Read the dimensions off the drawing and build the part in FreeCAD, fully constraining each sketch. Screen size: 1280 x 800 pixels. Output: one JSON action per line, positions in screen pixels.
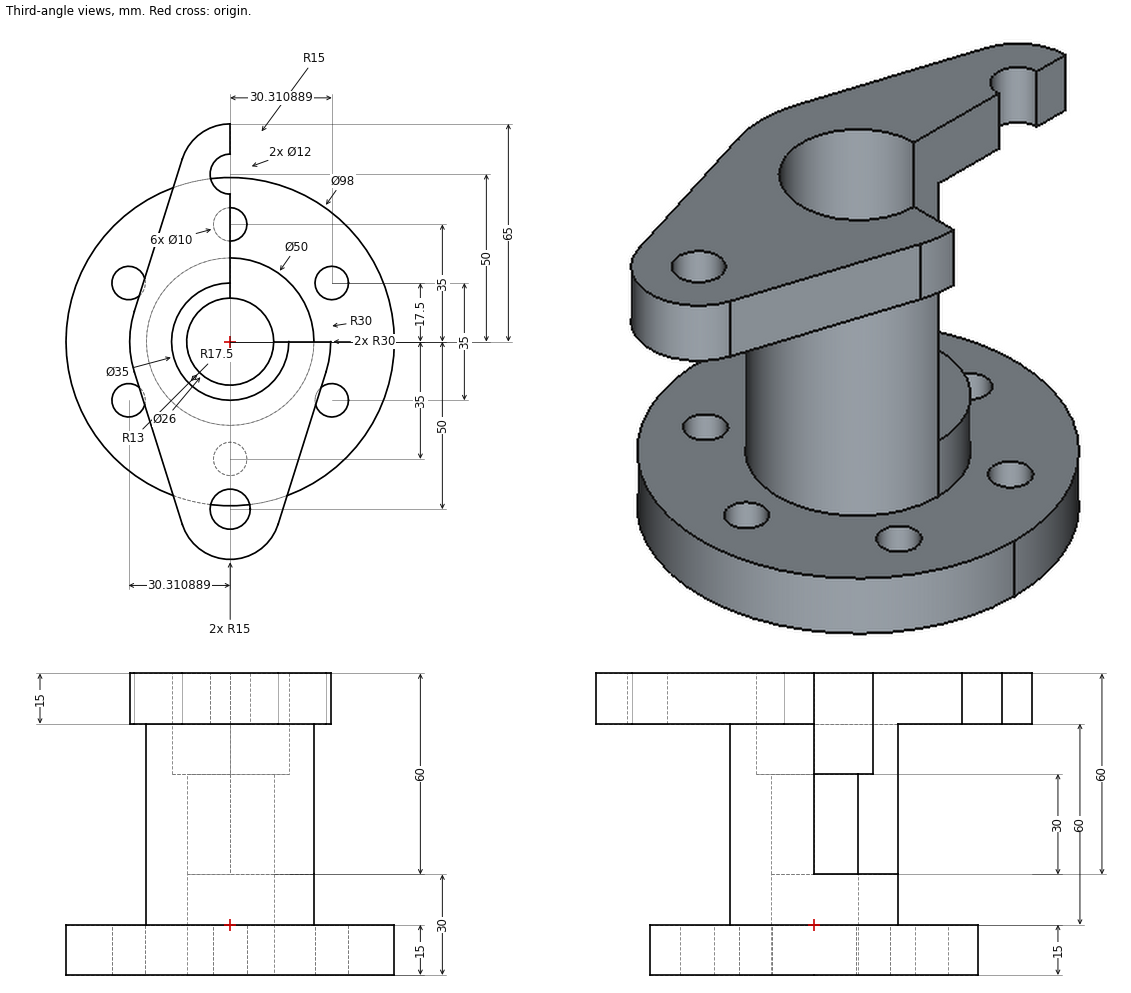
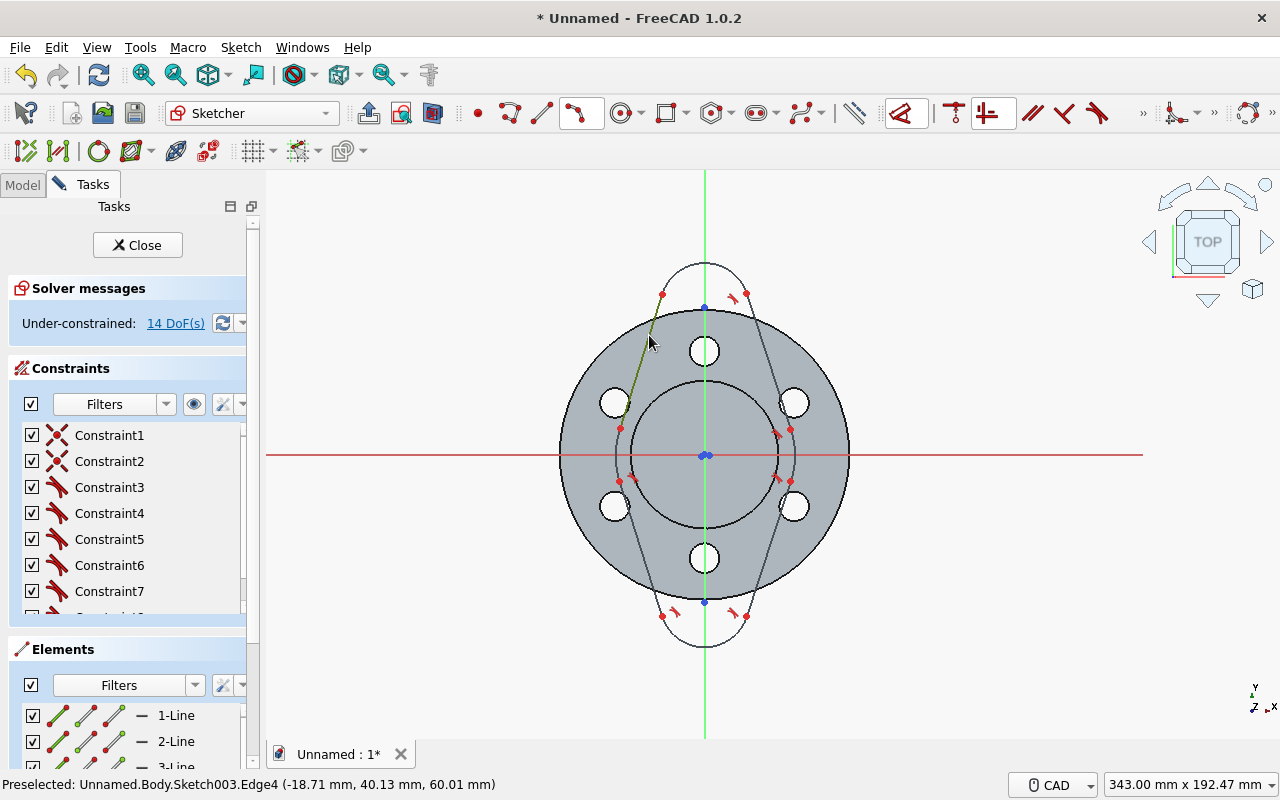
{"action": "left_click", "coordinate": [726, 268]}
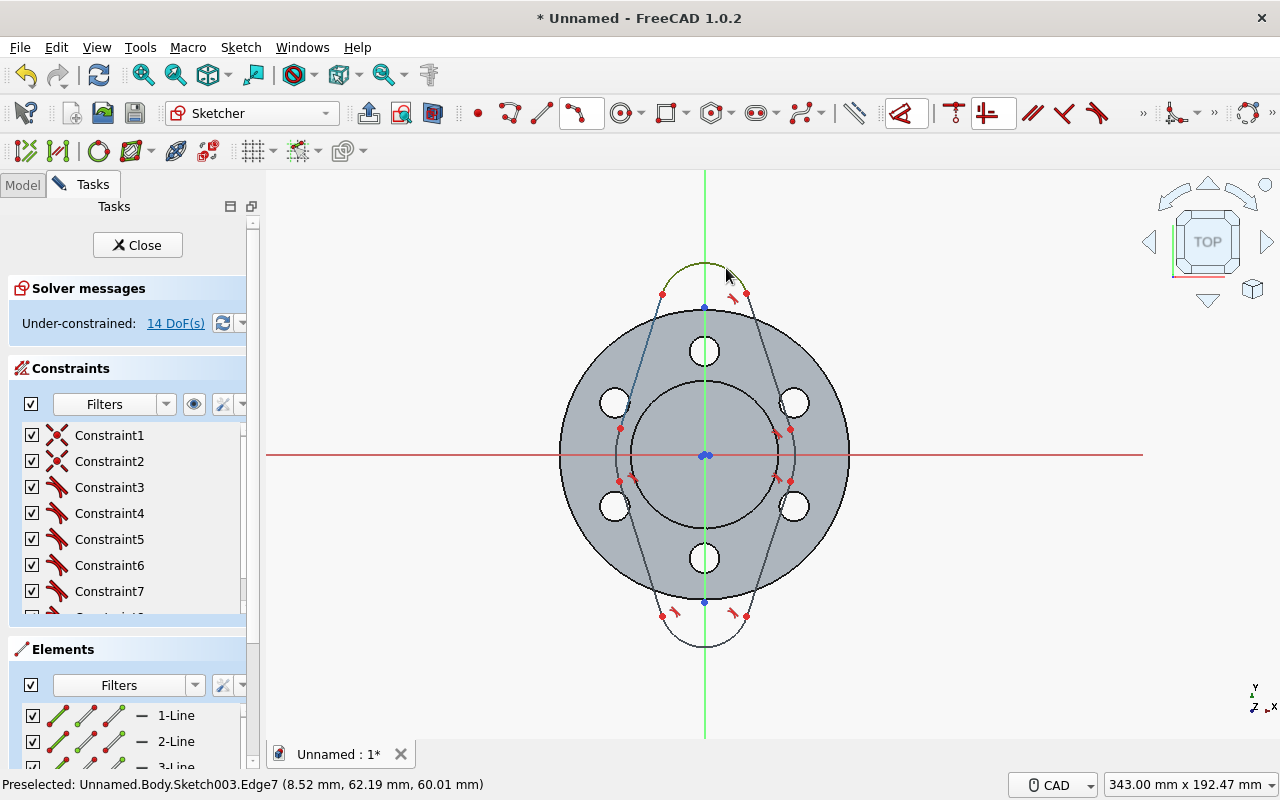
{"action": "left_click", "coordinate": [1098, 114]}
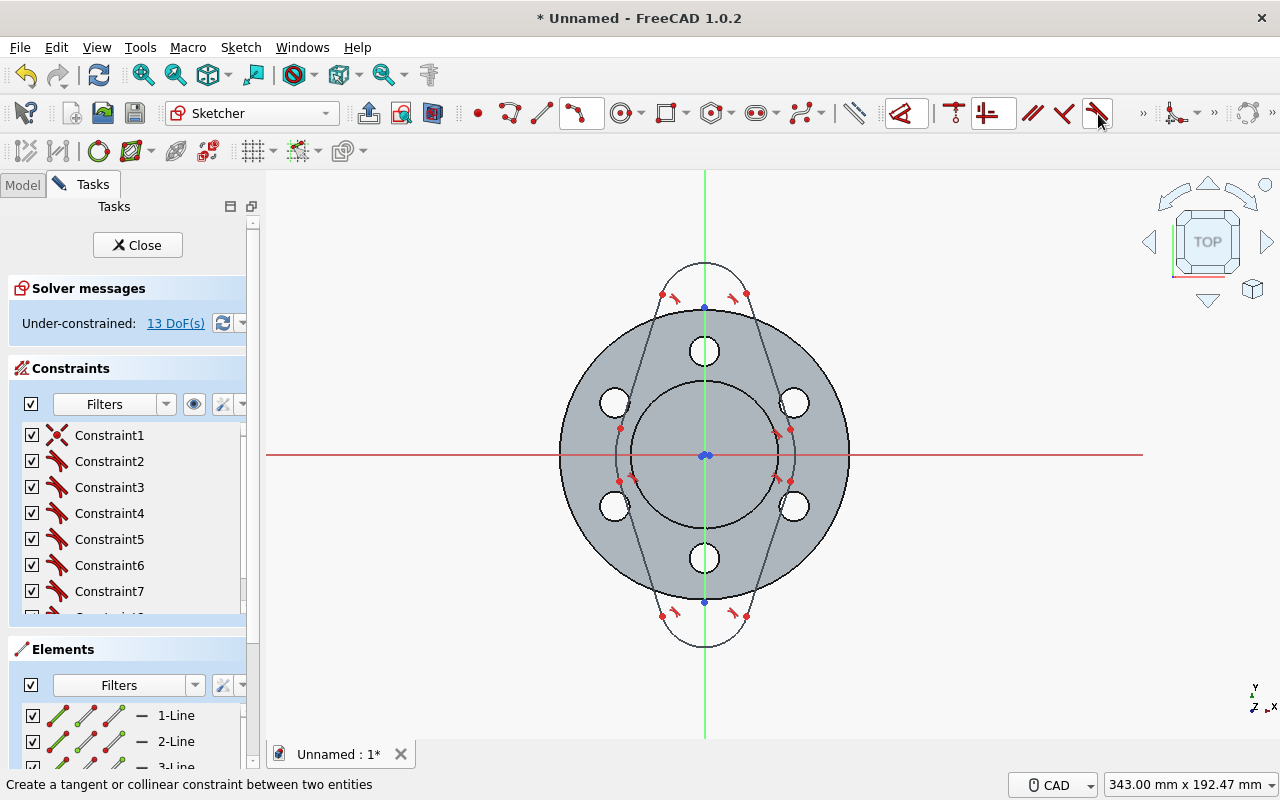
{"action": "left_click", "coordinate": [649, 335]}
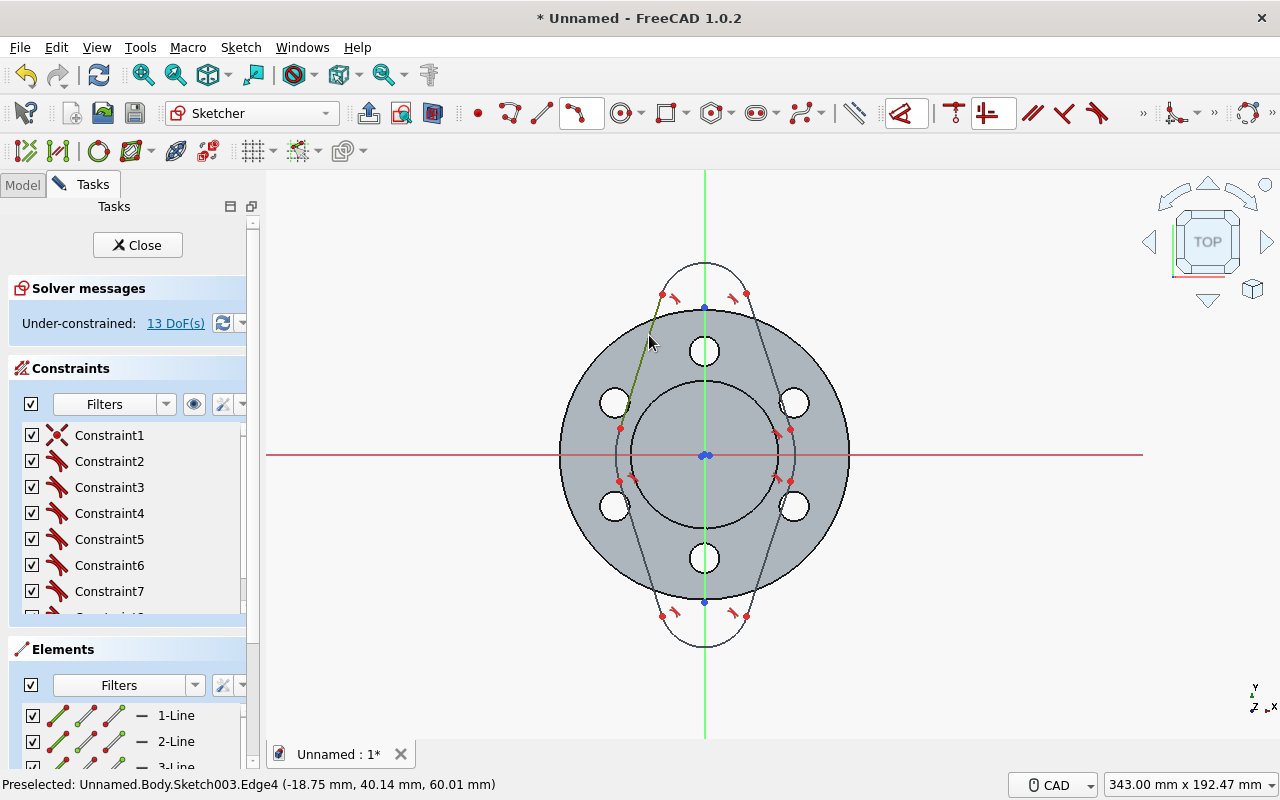
{"action": "scroll", "coordinate": [617, 445], "scroll_direction": "up", "scroll_amount": 2}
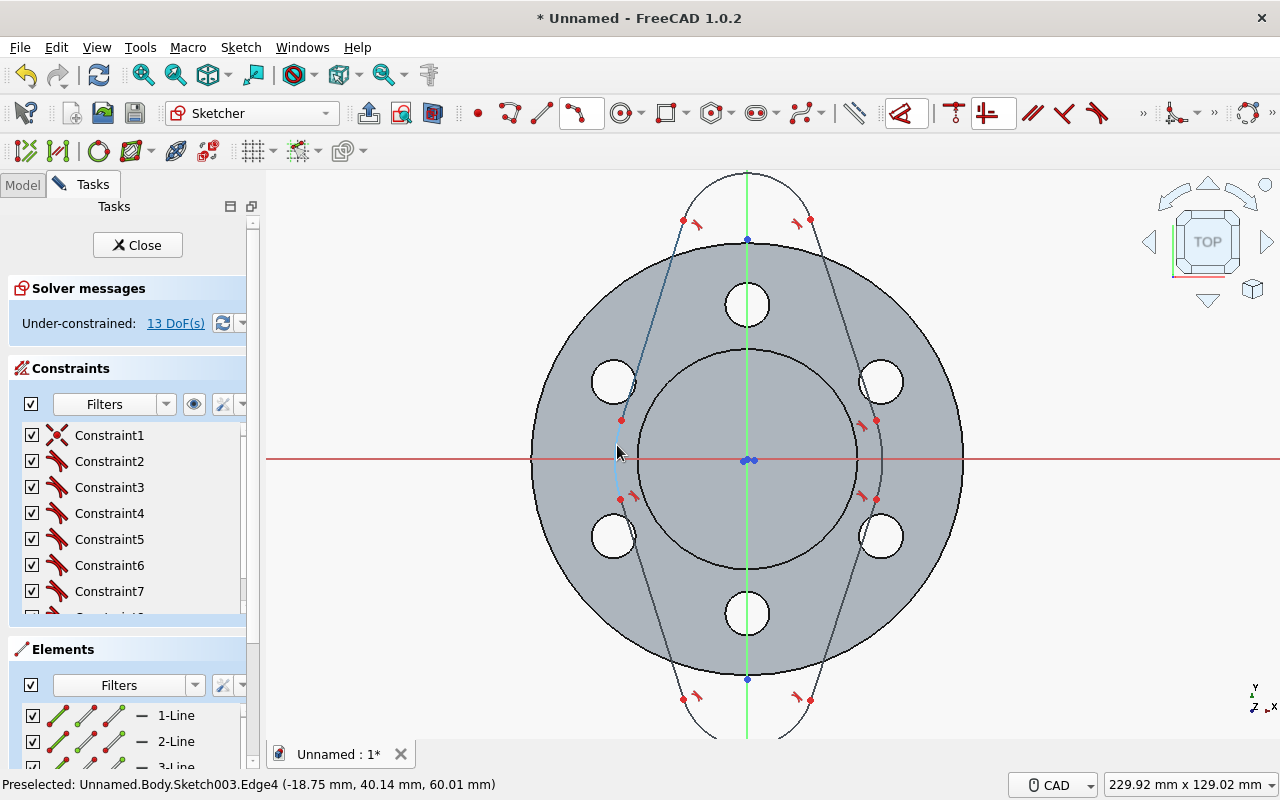
{"action": "left_click", "coordinate": [616, 444]}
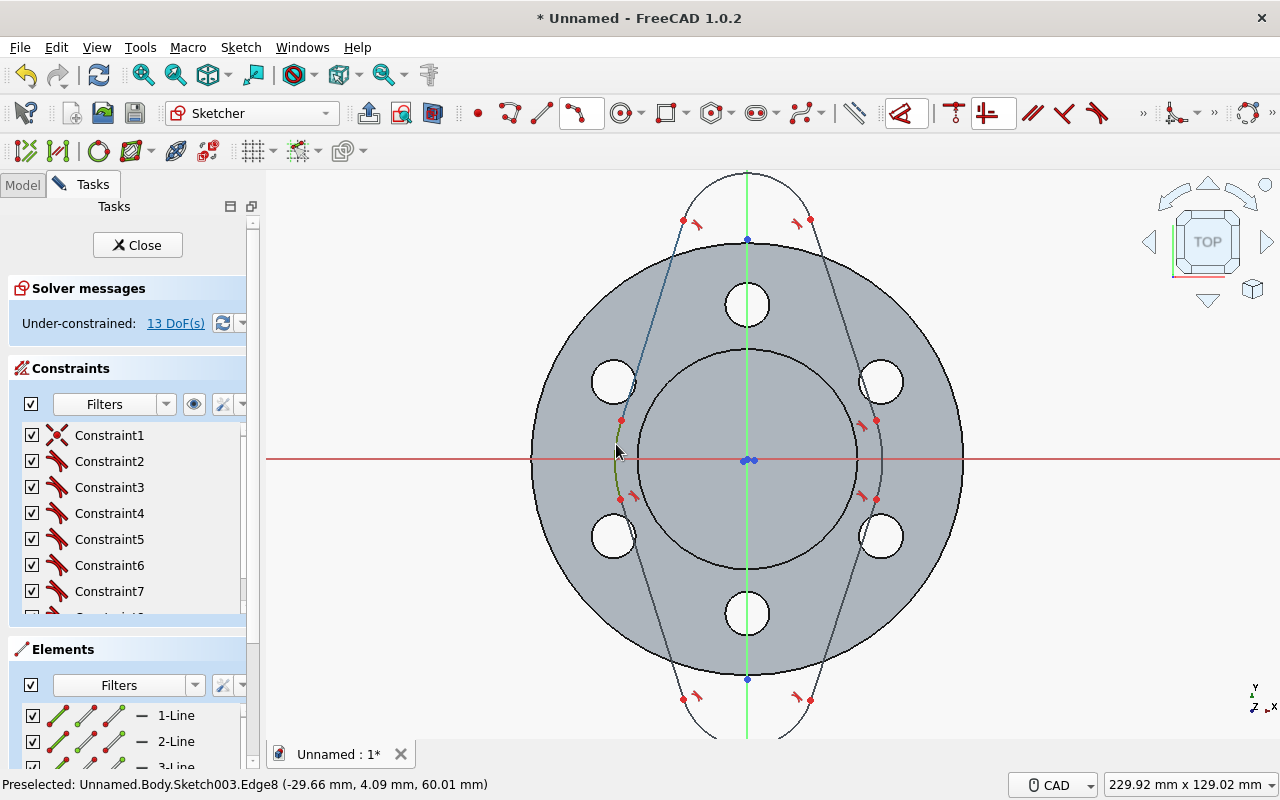
{"action": "left_click", "coordinate": [1098, 114]}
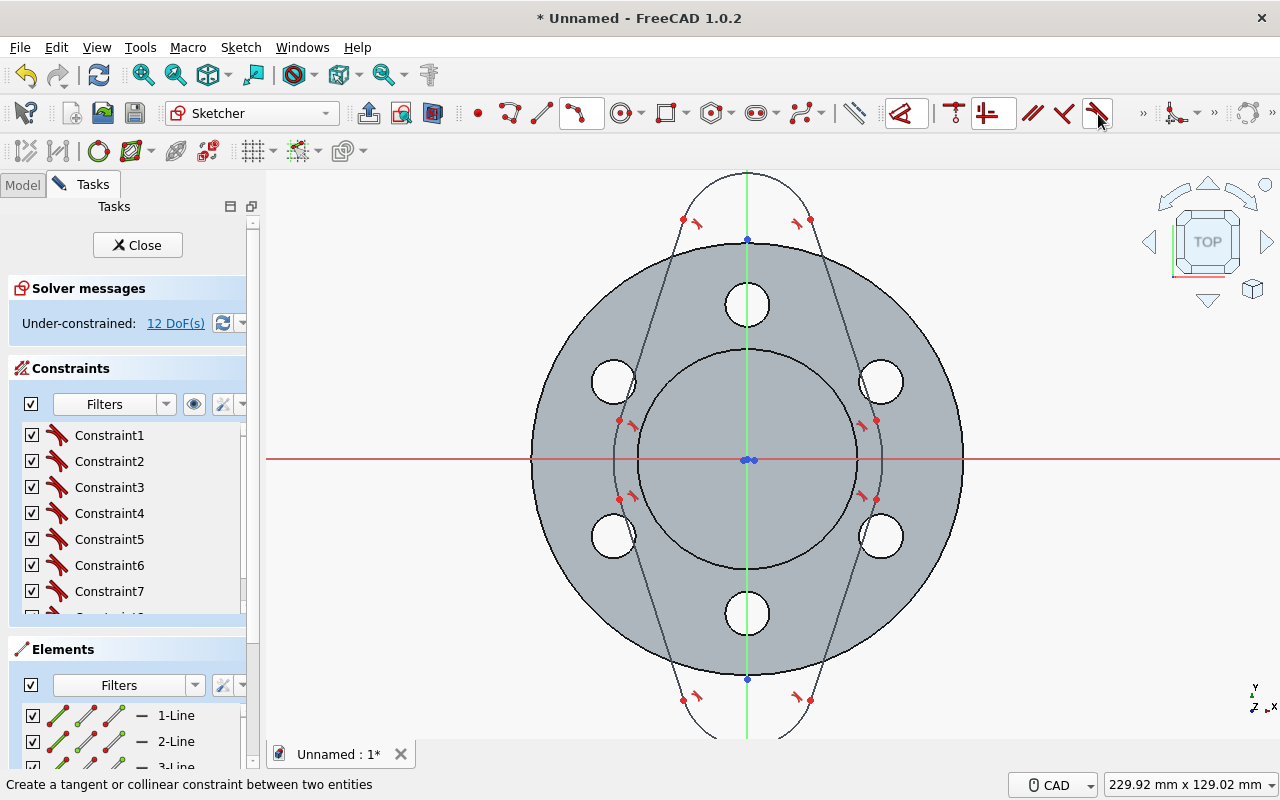
{"action": "left_click", "coordinate": [881, 476]}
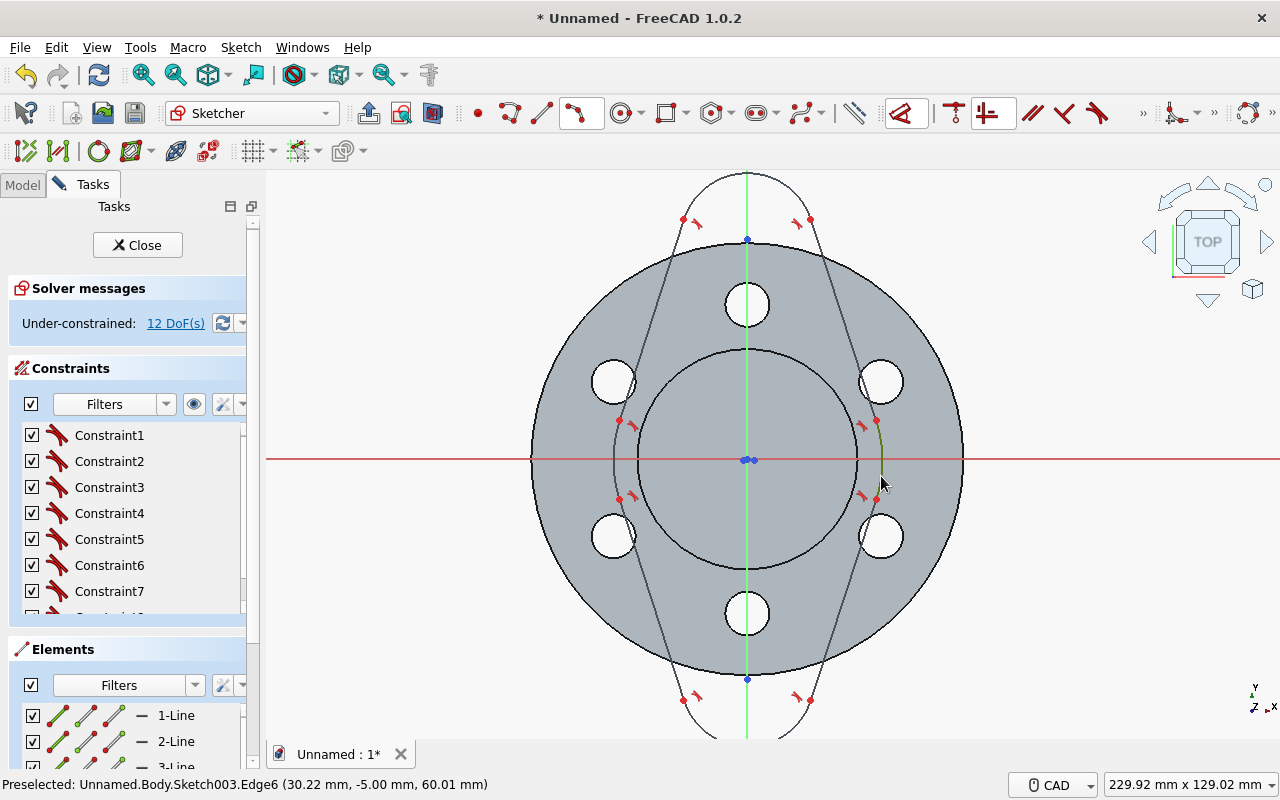
{"action": "left_click", "coordinate": [615, 444]}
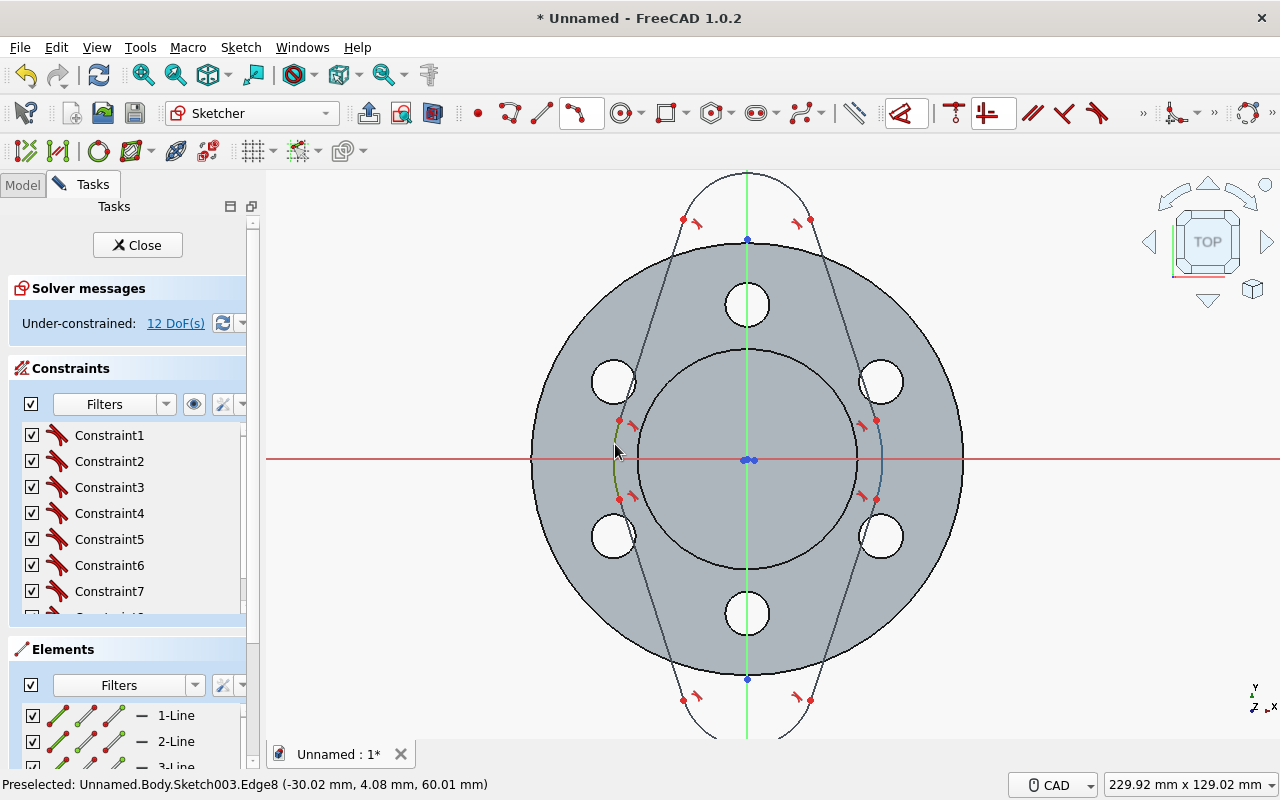
{"action": "left_click", "coordinate": [954, 114]}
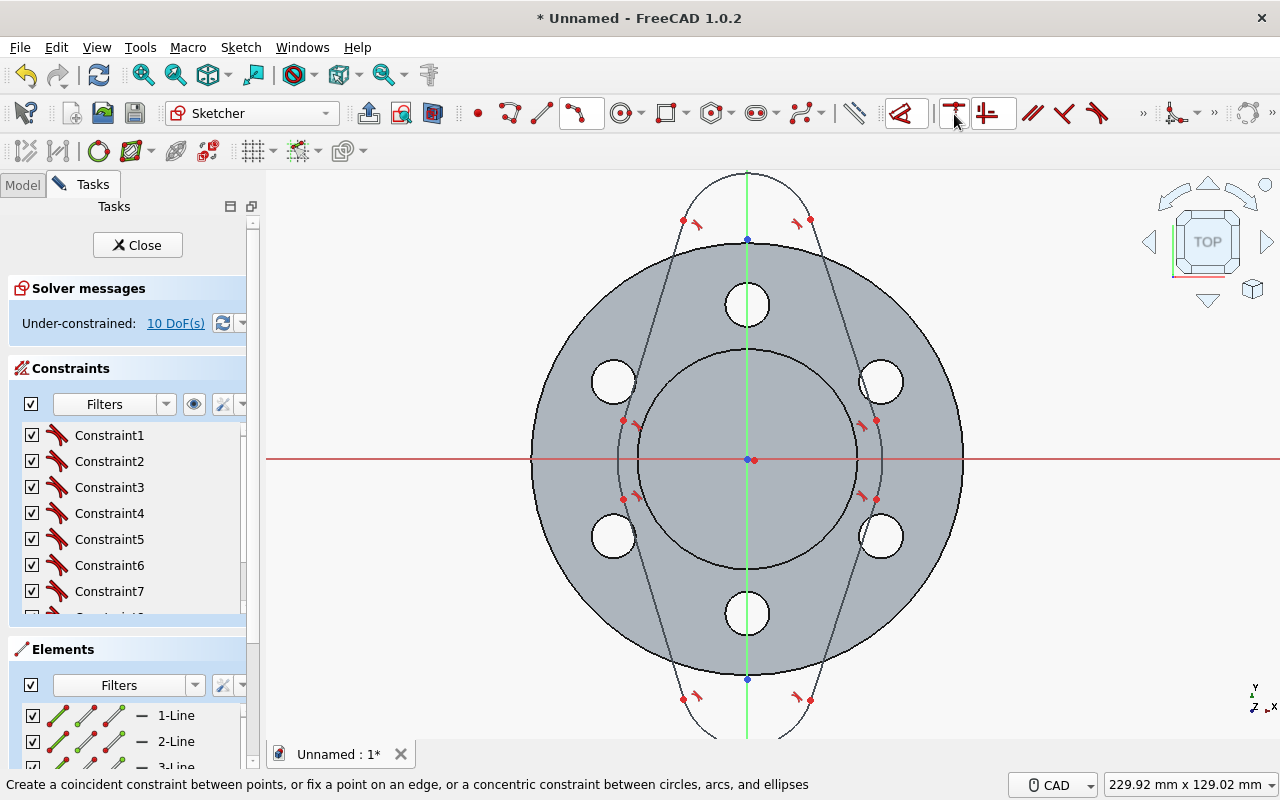
{"action": "left_click_drag", "start_coordinate": [737, 449], "coordinate": [764, 470]}